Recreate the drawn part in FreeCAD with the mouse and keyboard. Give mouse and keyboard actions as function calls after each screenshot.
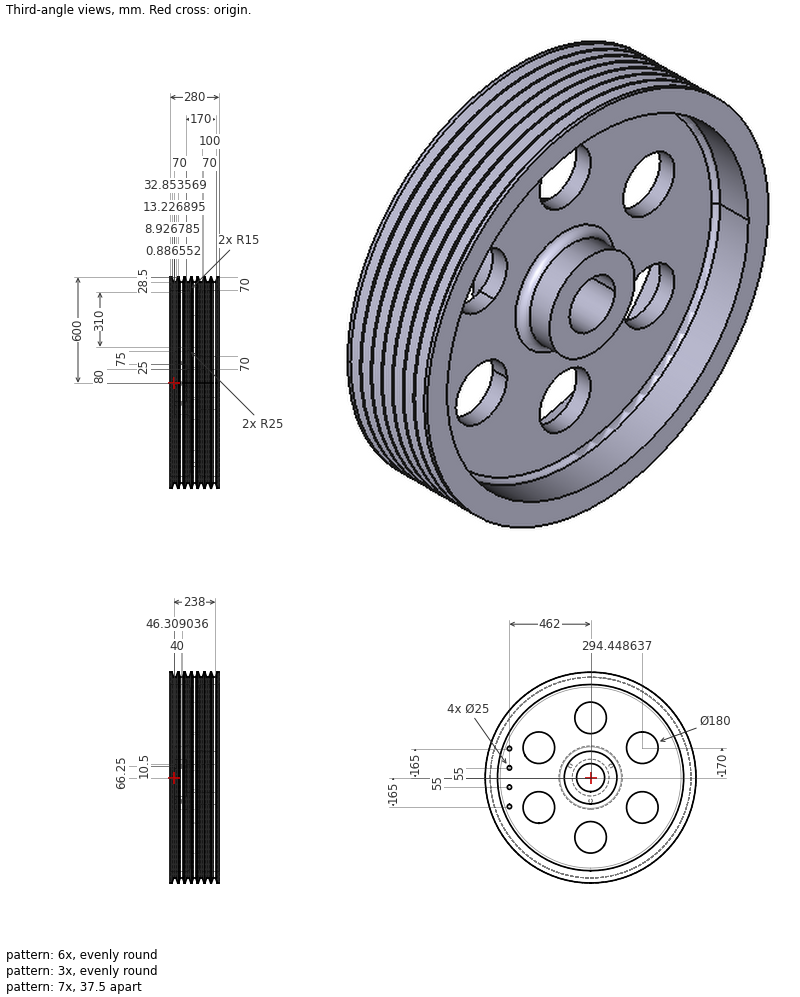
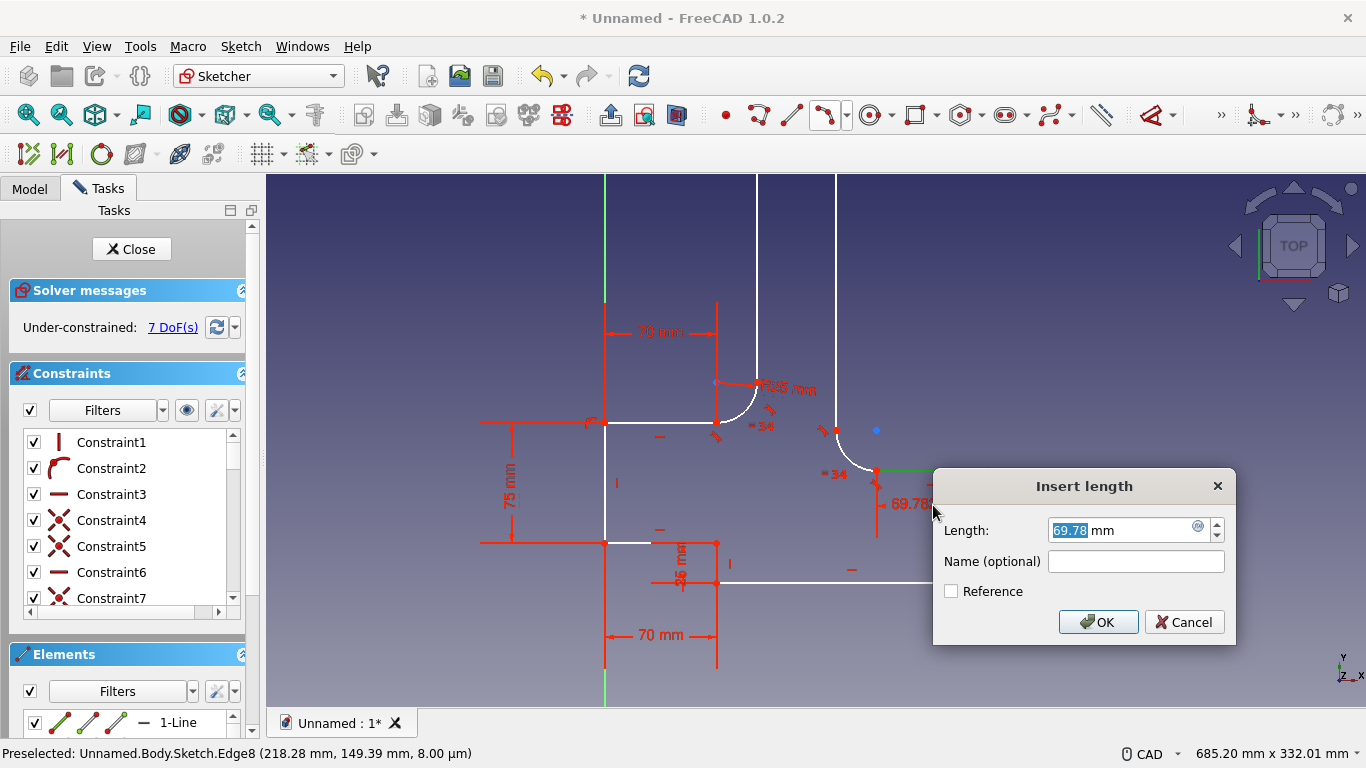
text(70)
key(Return)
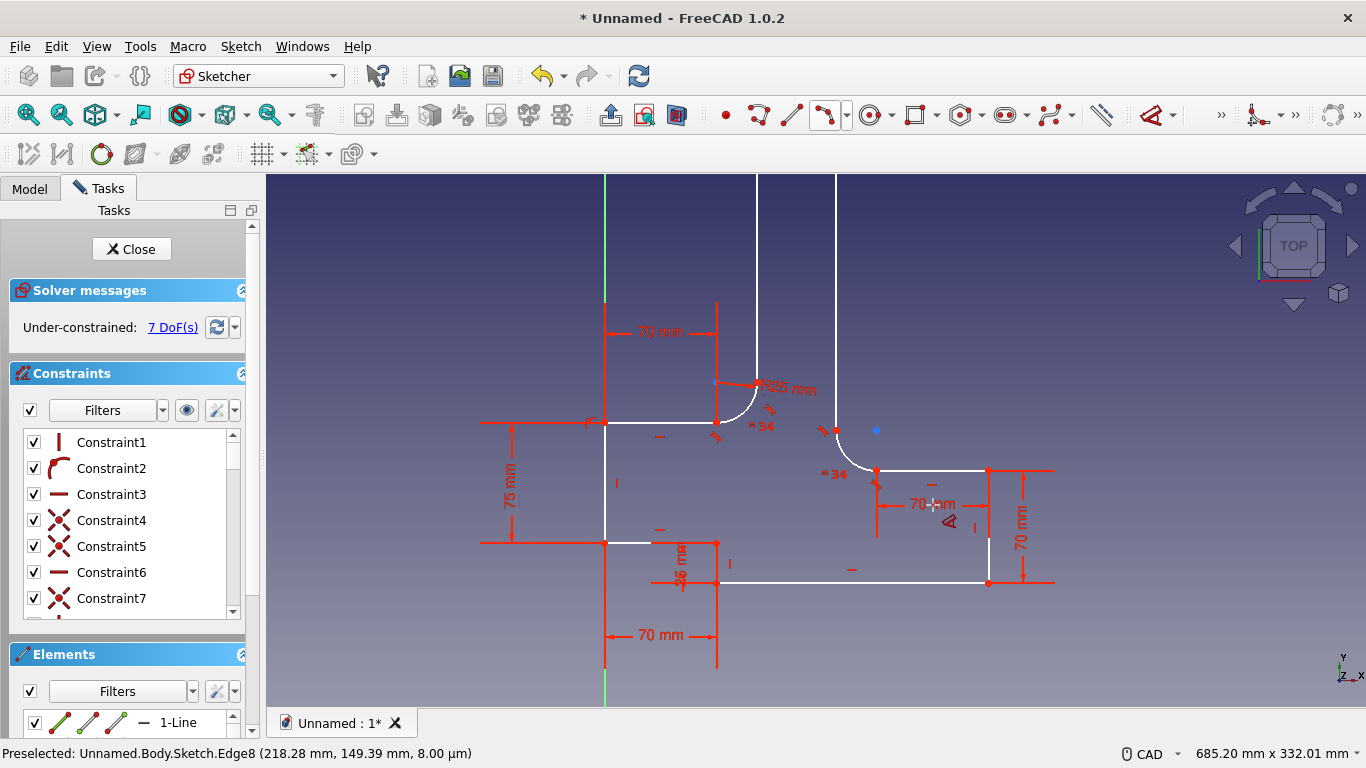
scroll(719, 564, down, 5)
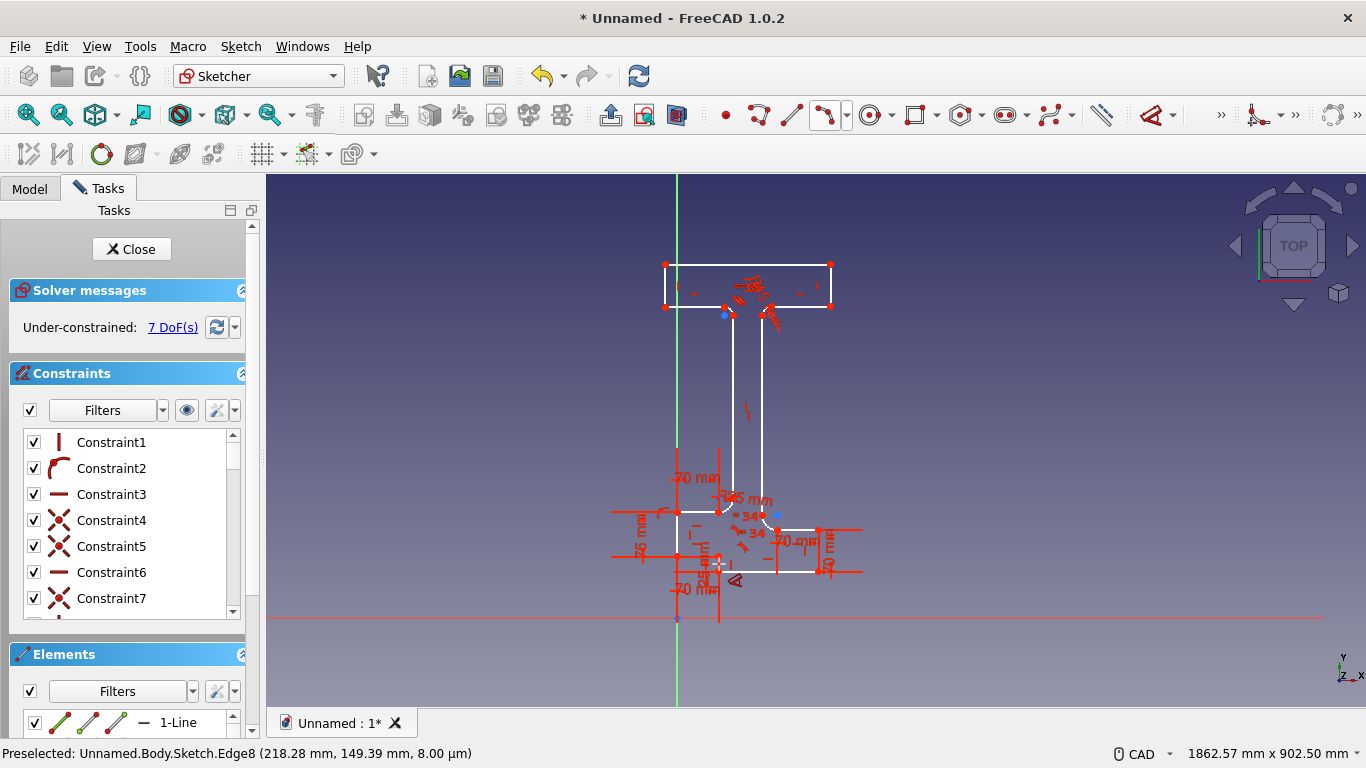
click(831, 294)
click(865, 286)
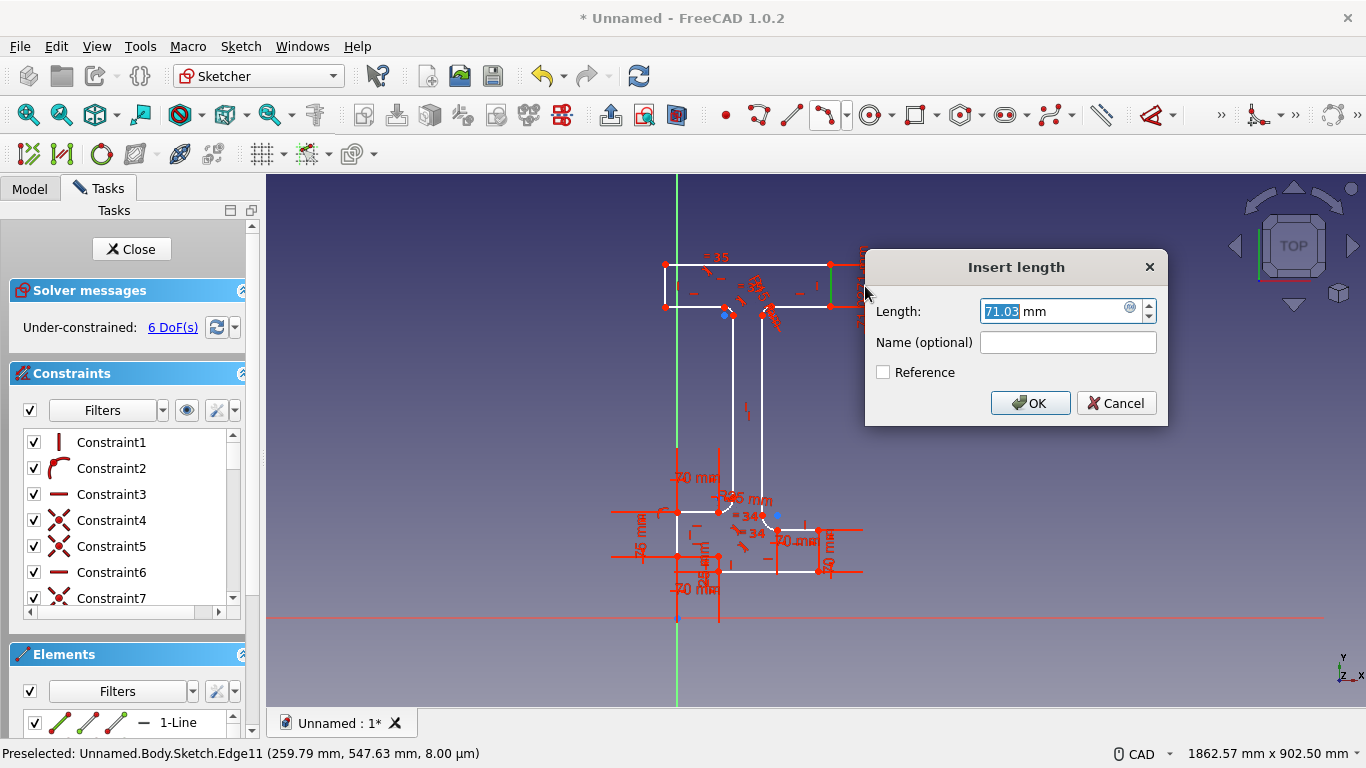
text(70)
key(Return)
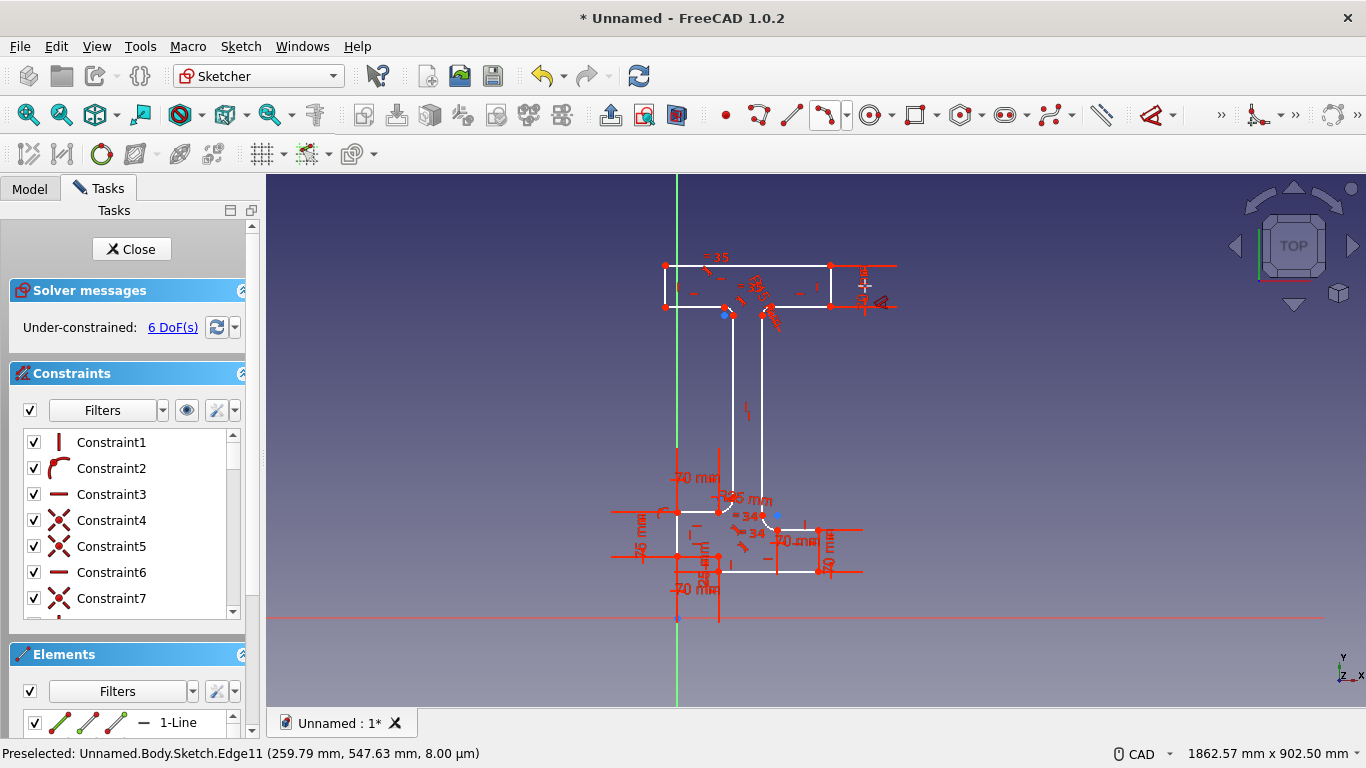
click(665, 278)
click(631, 286)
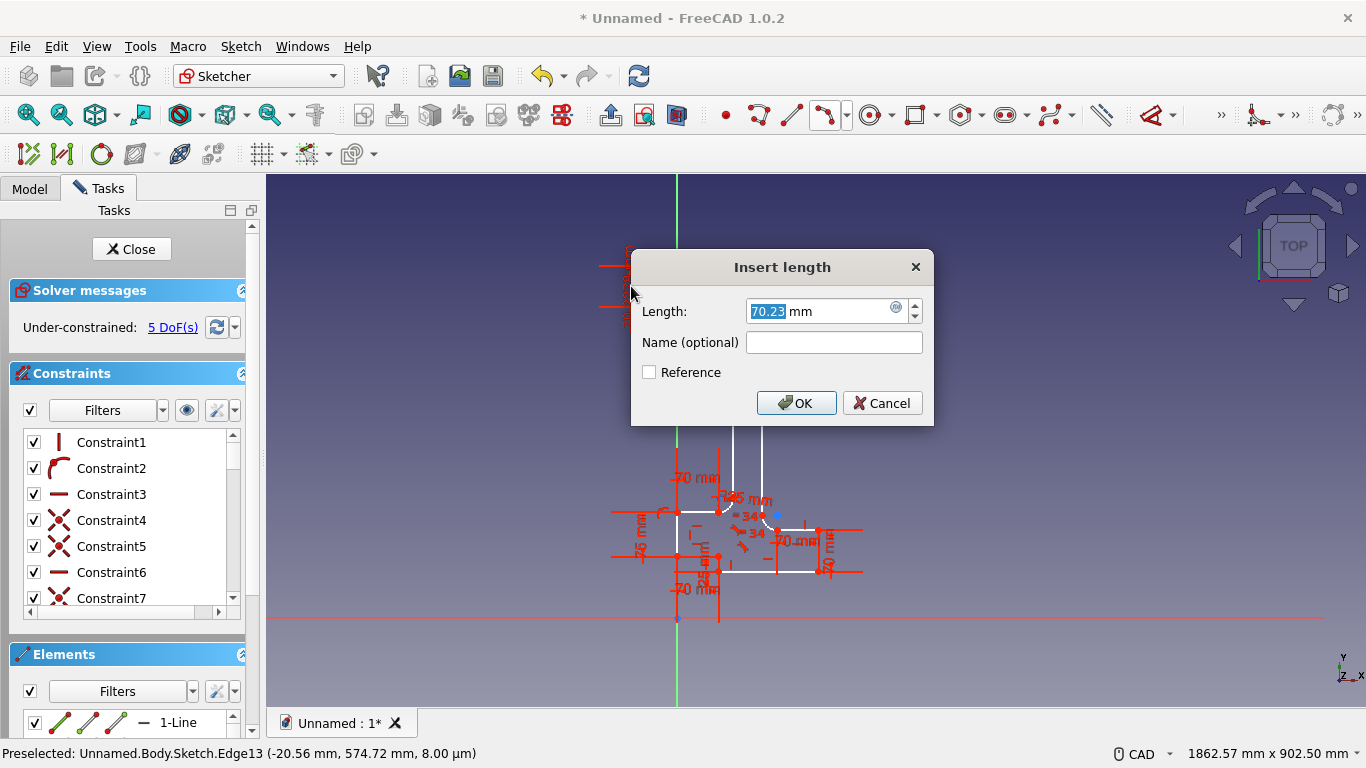
text(70)
key(Return)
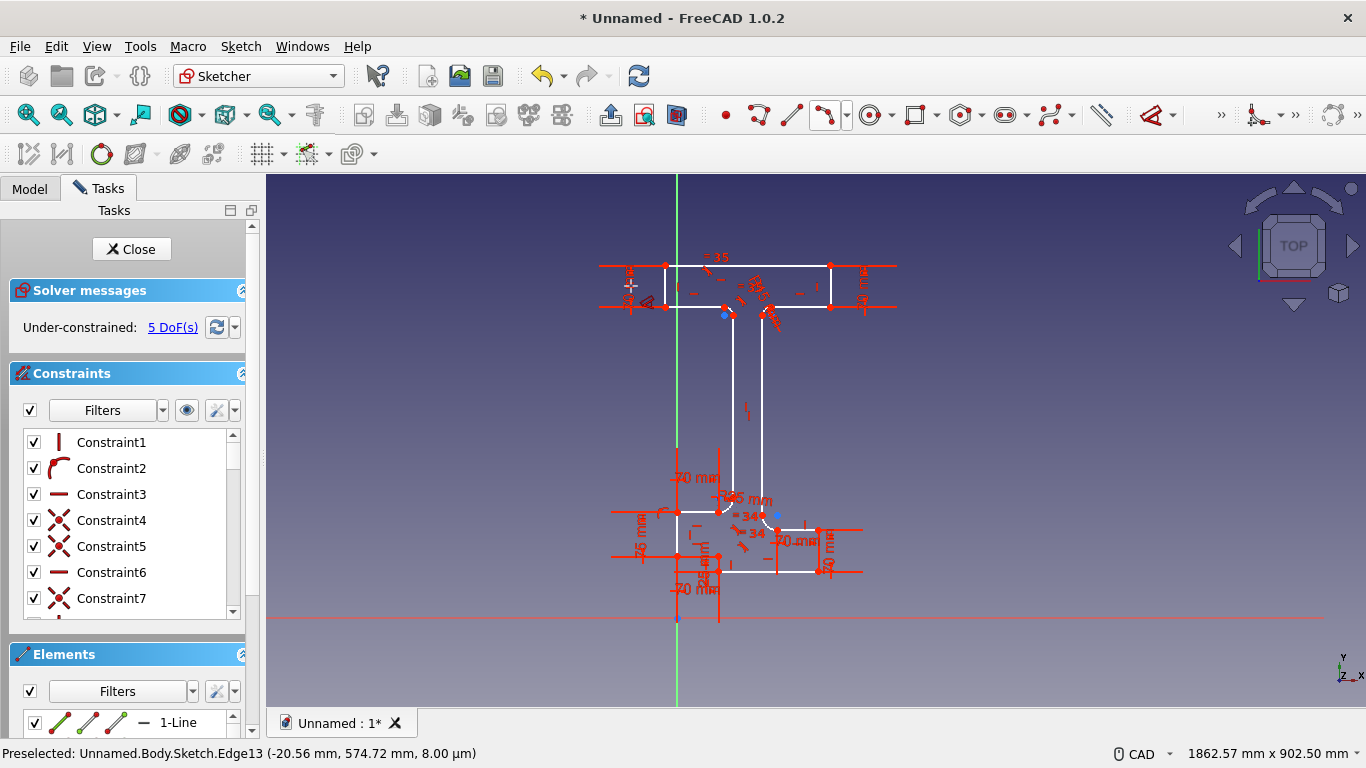
click(733, 370)
click(699, 407)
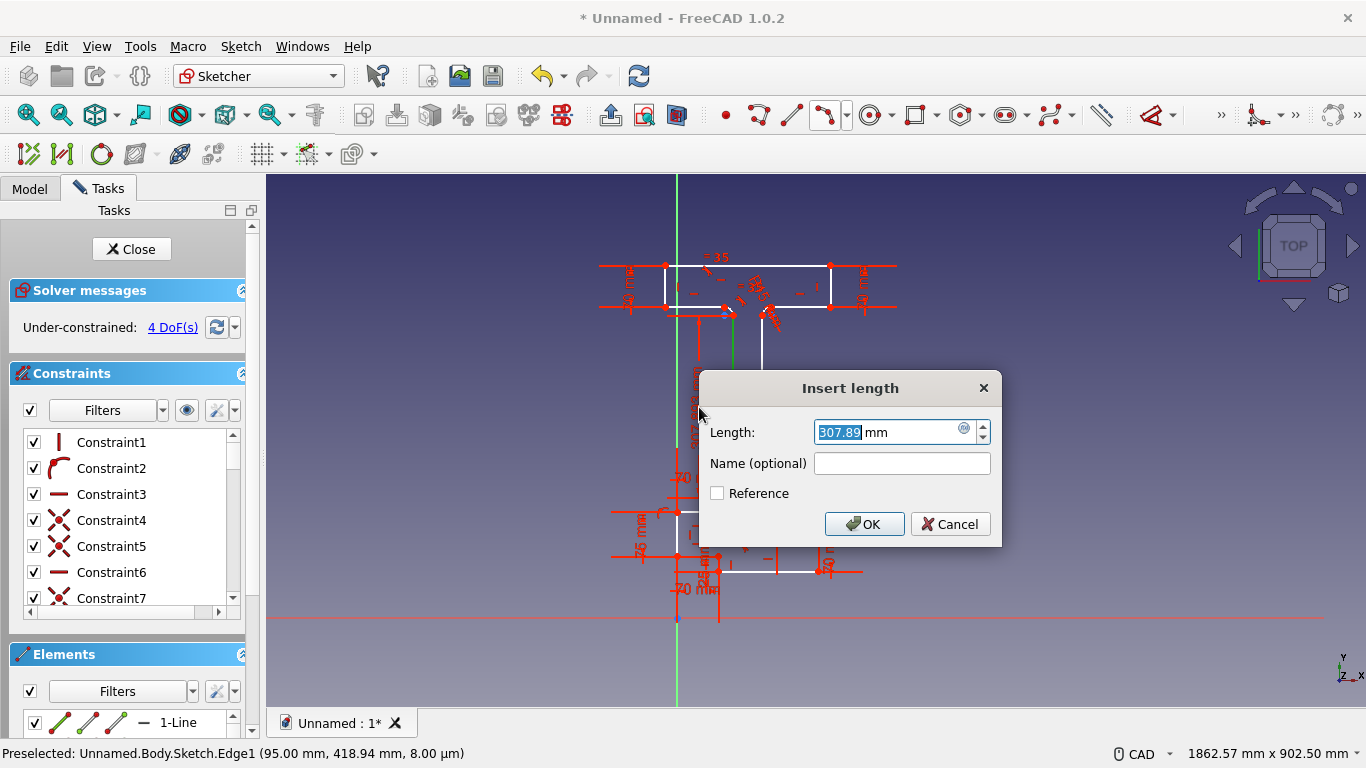
text(310)
key(Return)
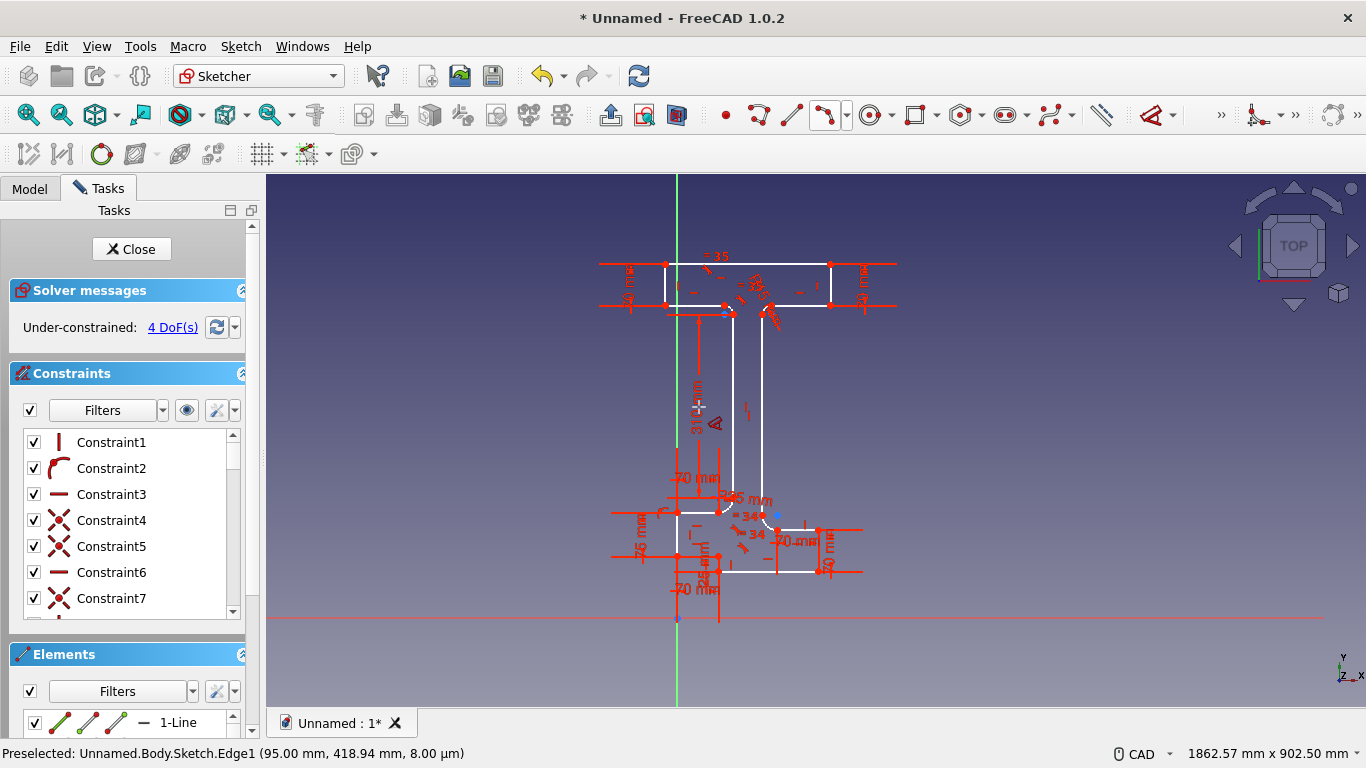
click(749, 572)
click(769, 654)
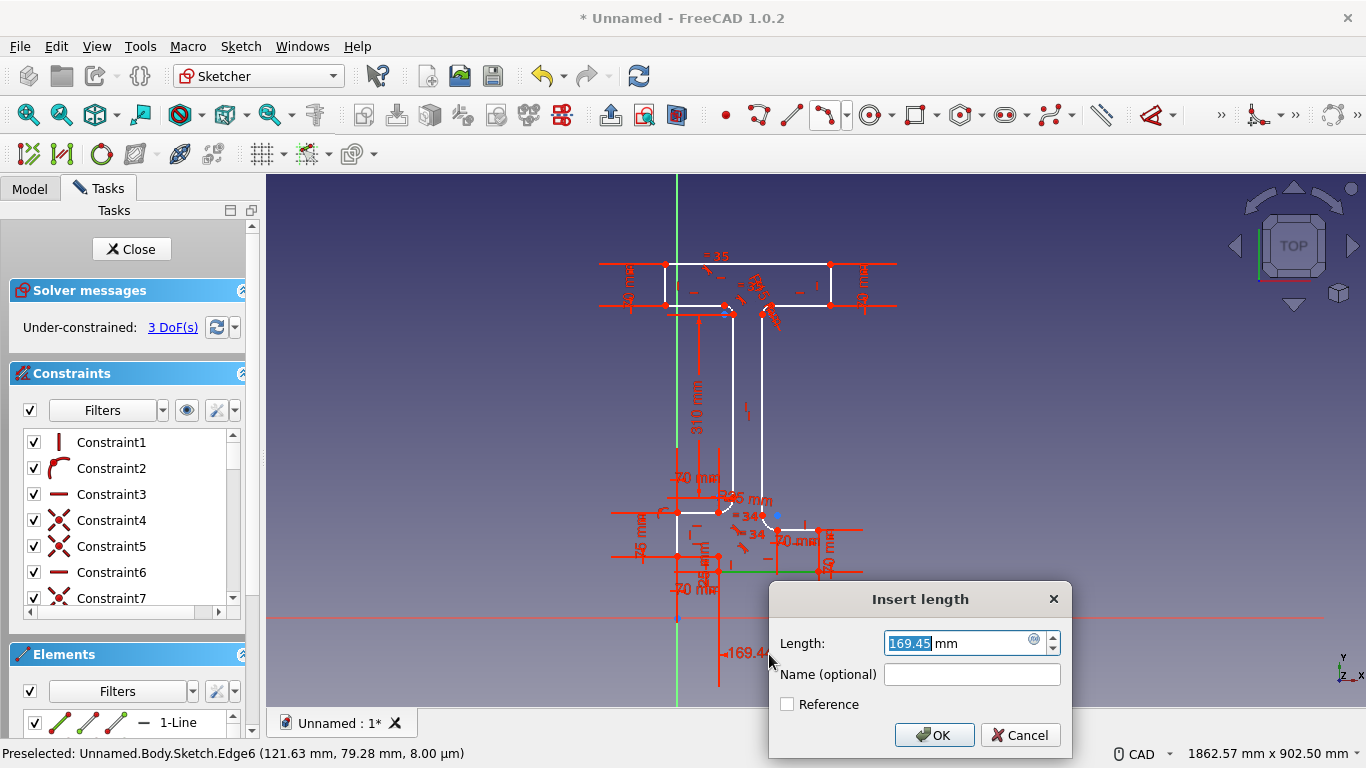
text(170)
key(Return)